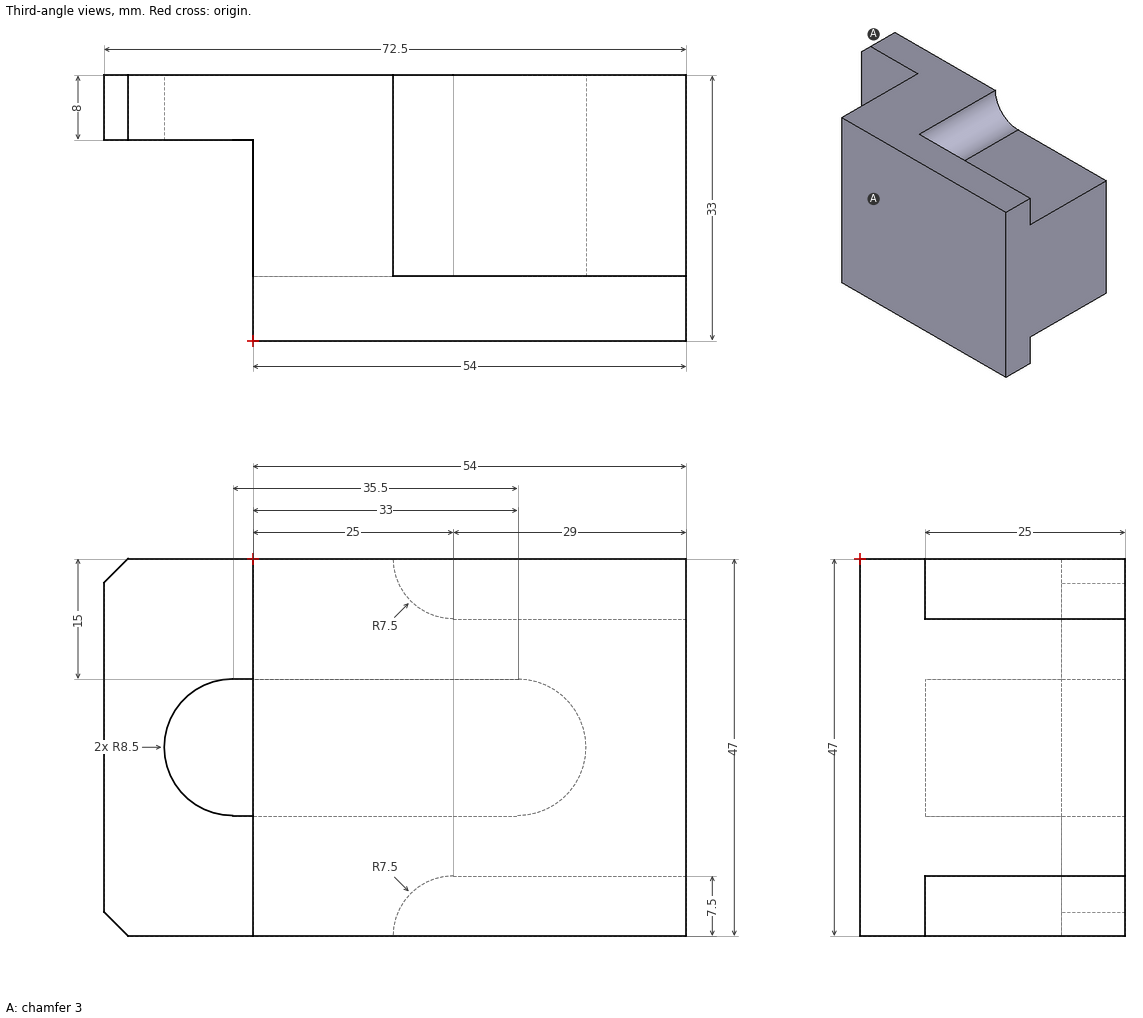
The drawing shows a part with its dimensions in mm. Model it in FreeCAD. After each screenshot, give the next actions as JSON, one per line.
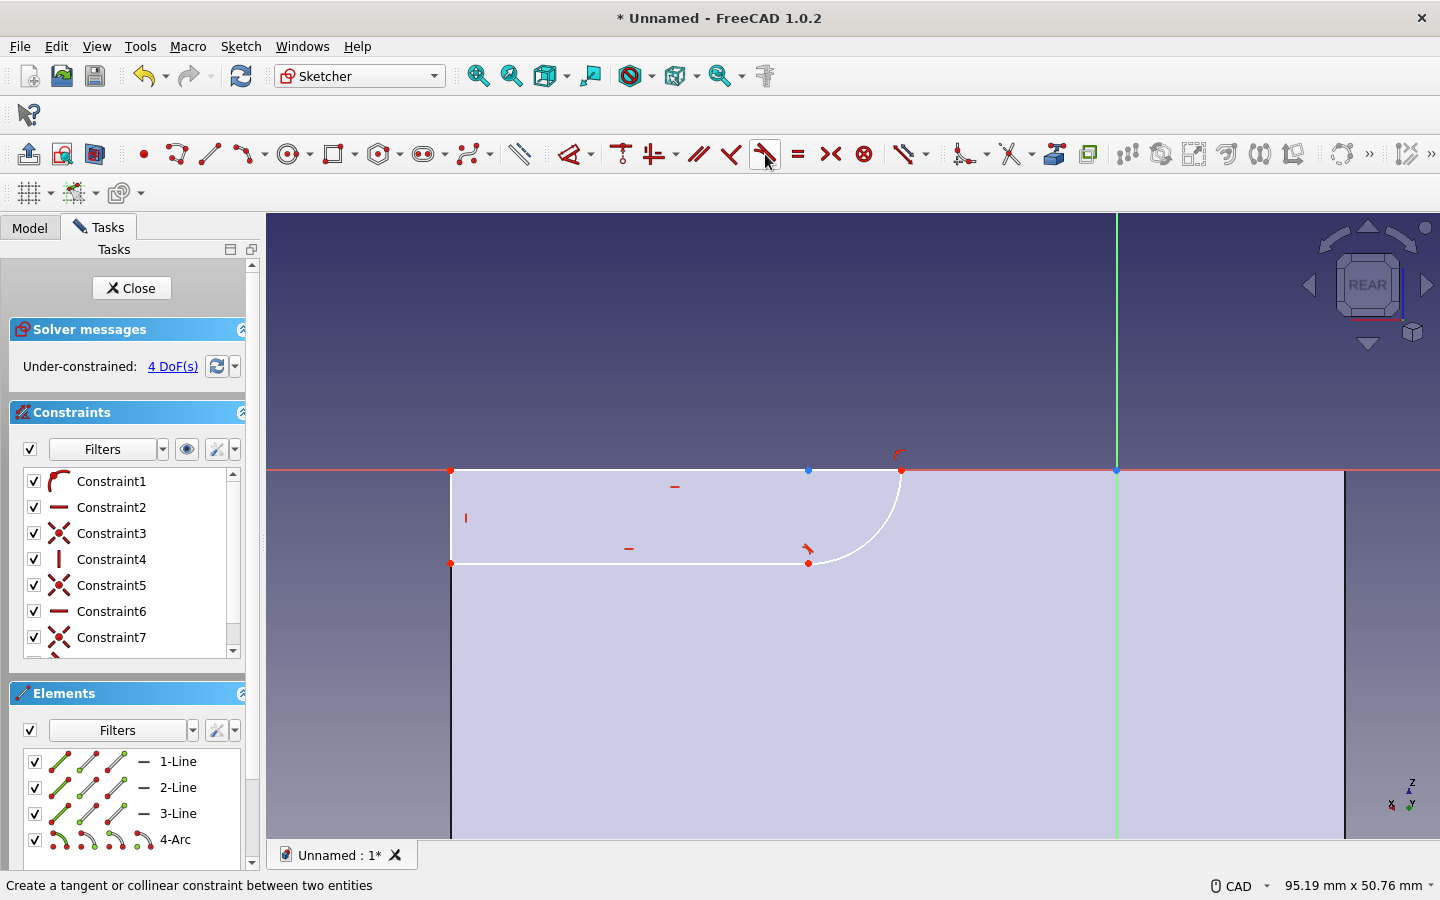
{"action": "left_click", "coordinate": [808, 471]}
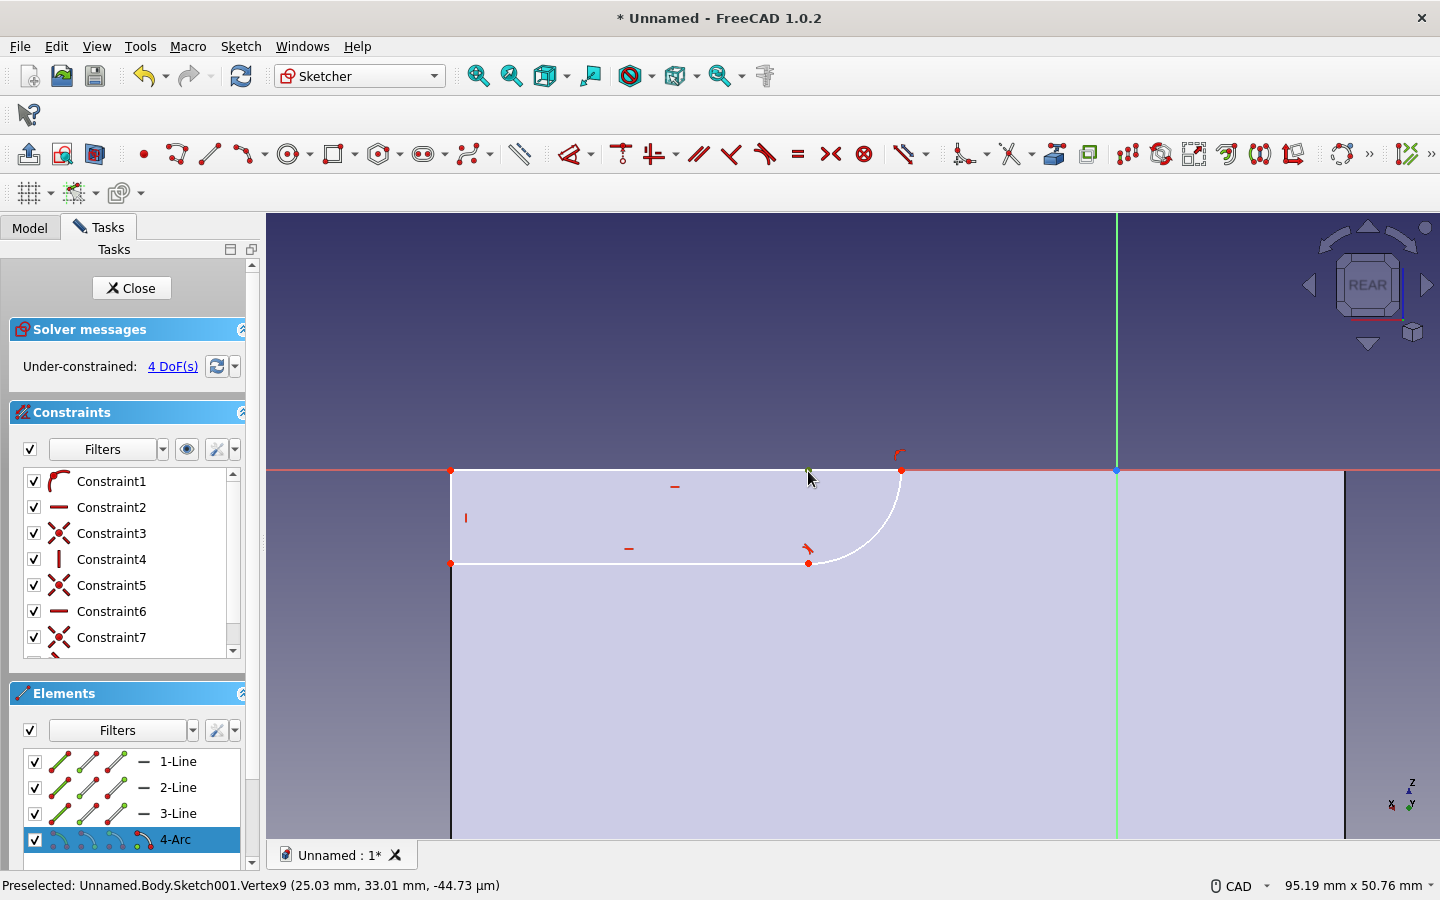
{"action": "left_click", "coordinate": [364, 470]}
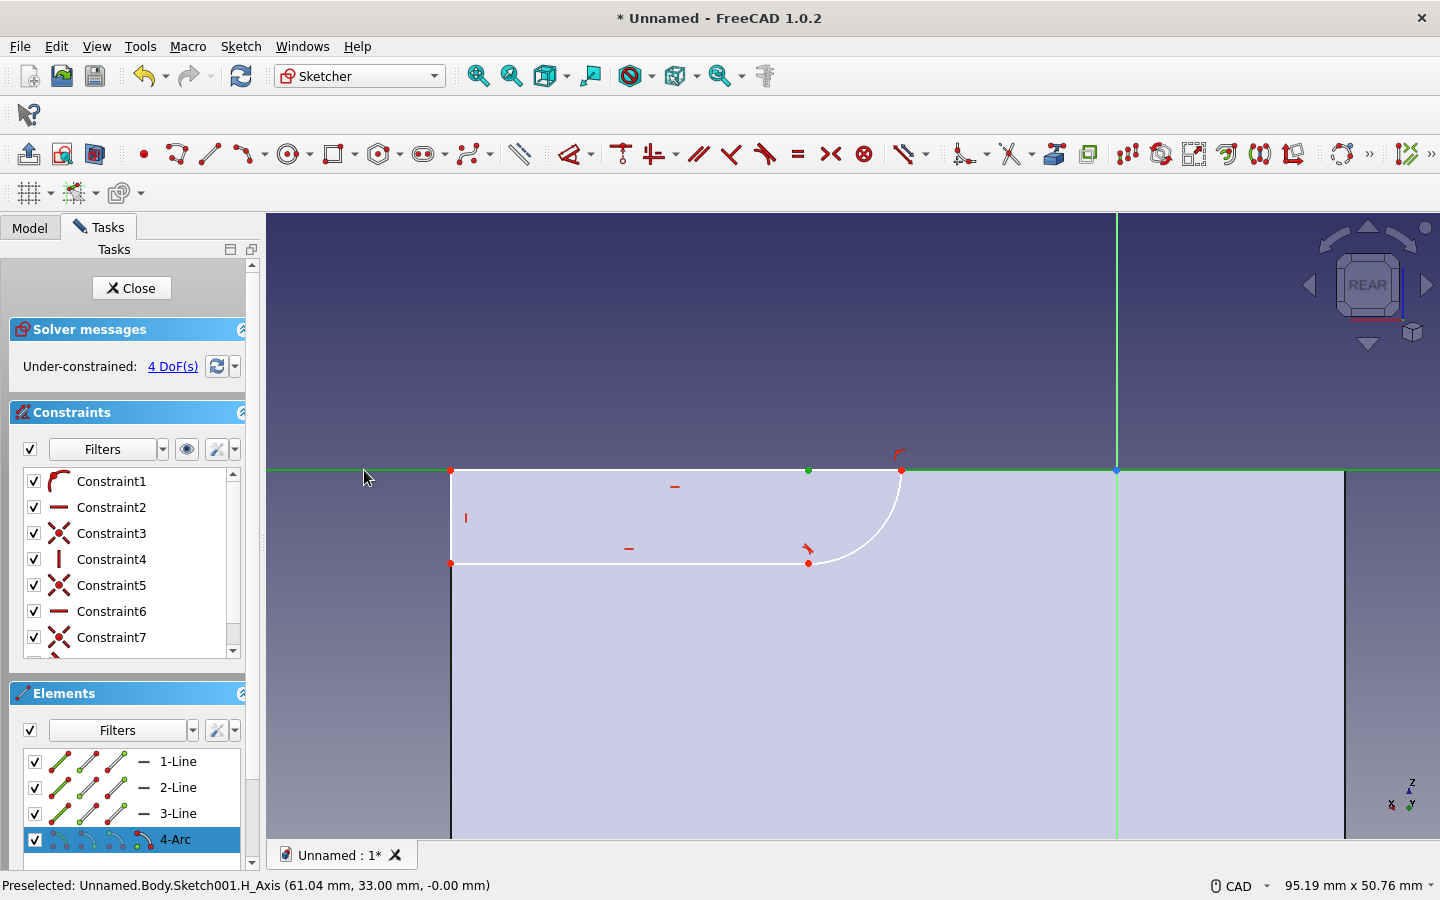
{"action": "key", "text": "c"}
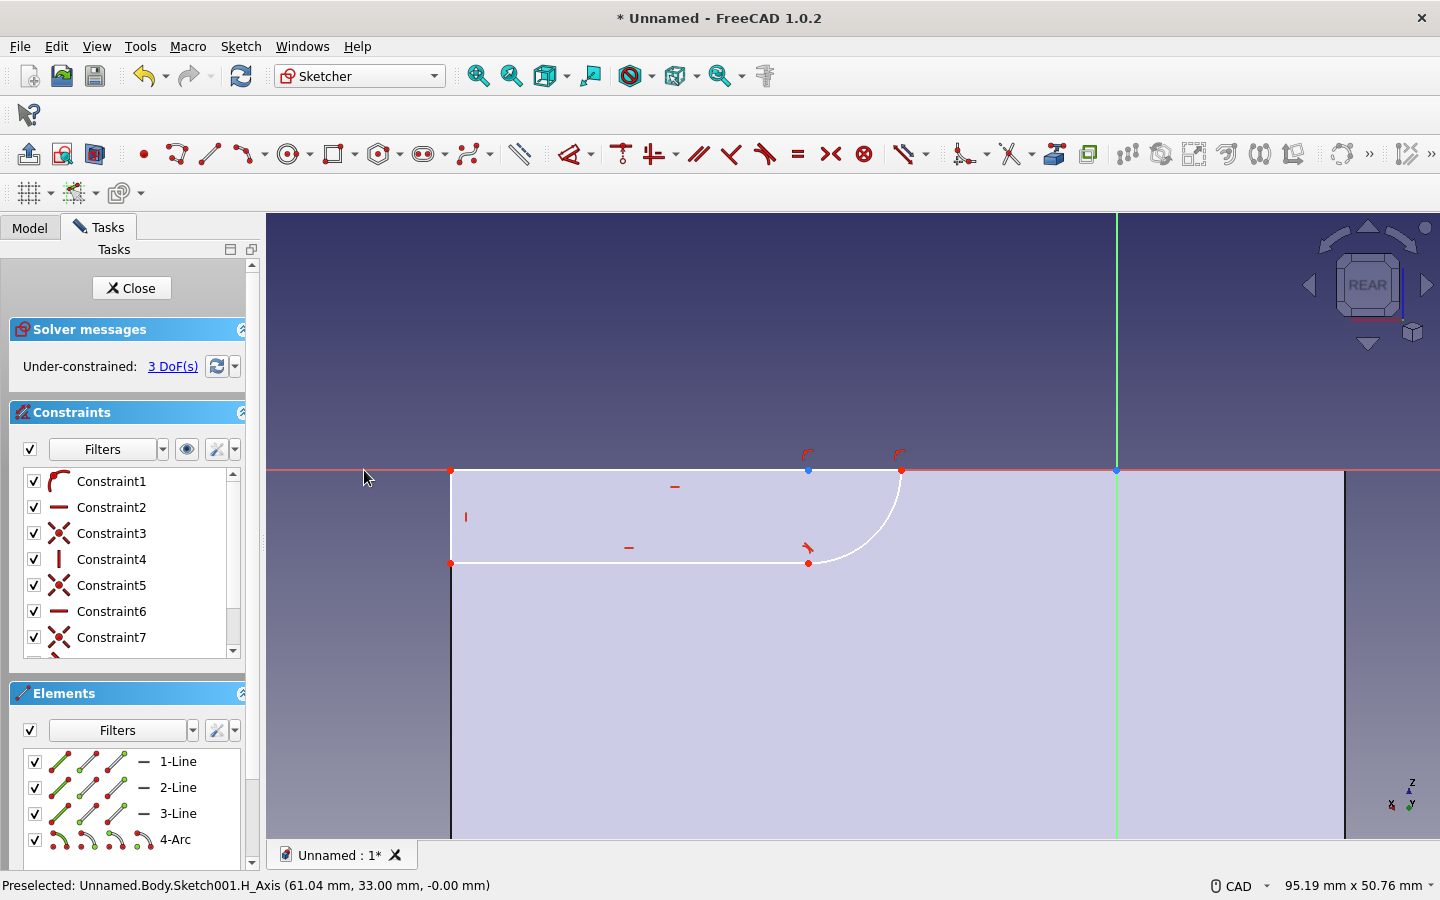
{"action": "key", "text": "d"}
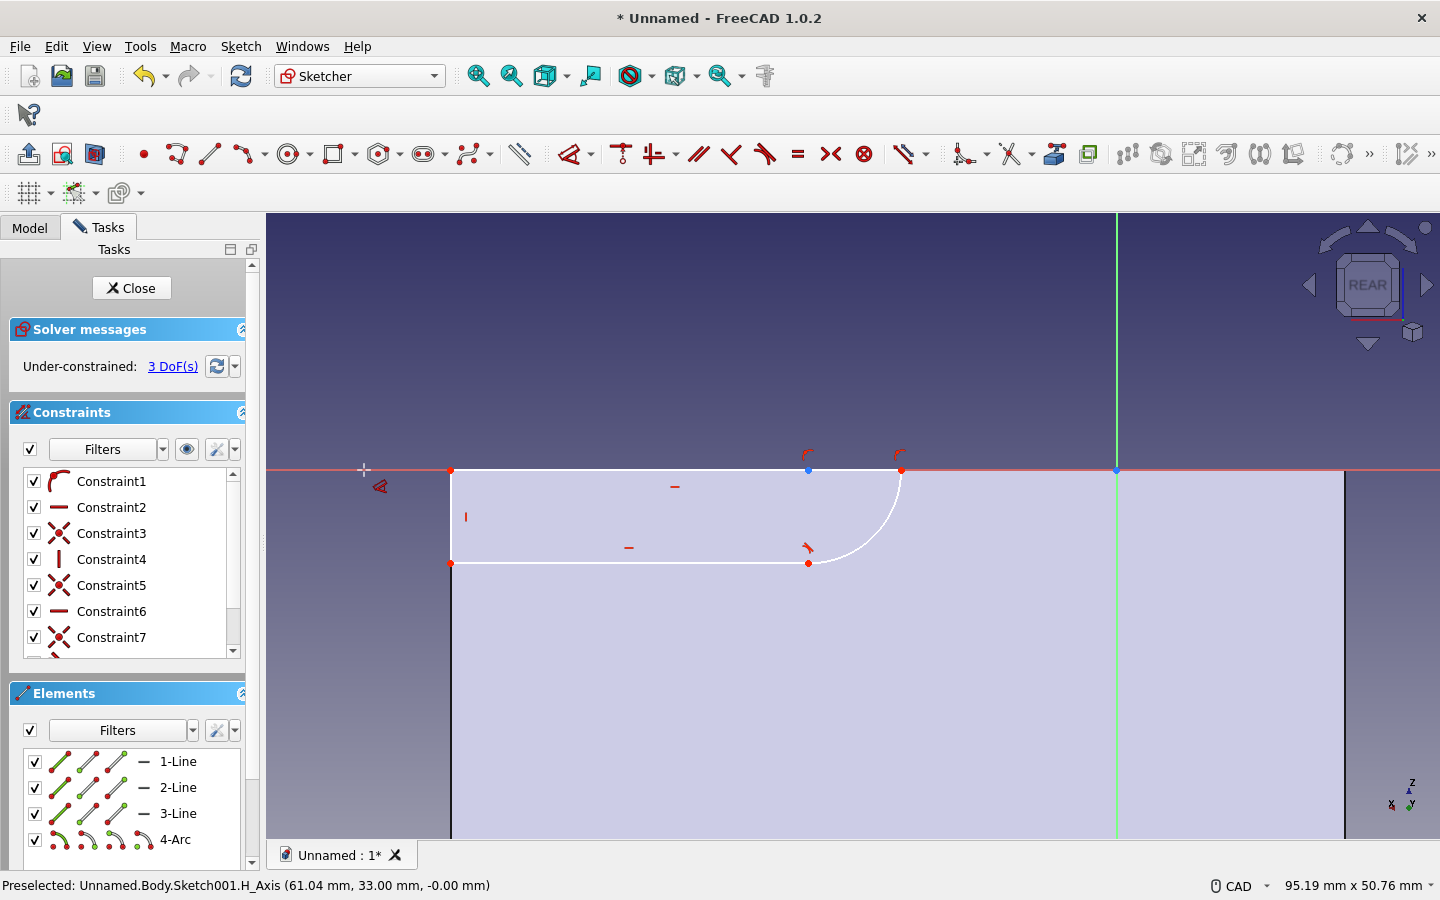
{"action": "left_click", "coordinate": [850, 553]}
{"action": "left_click", "coordinate": [865, 582]}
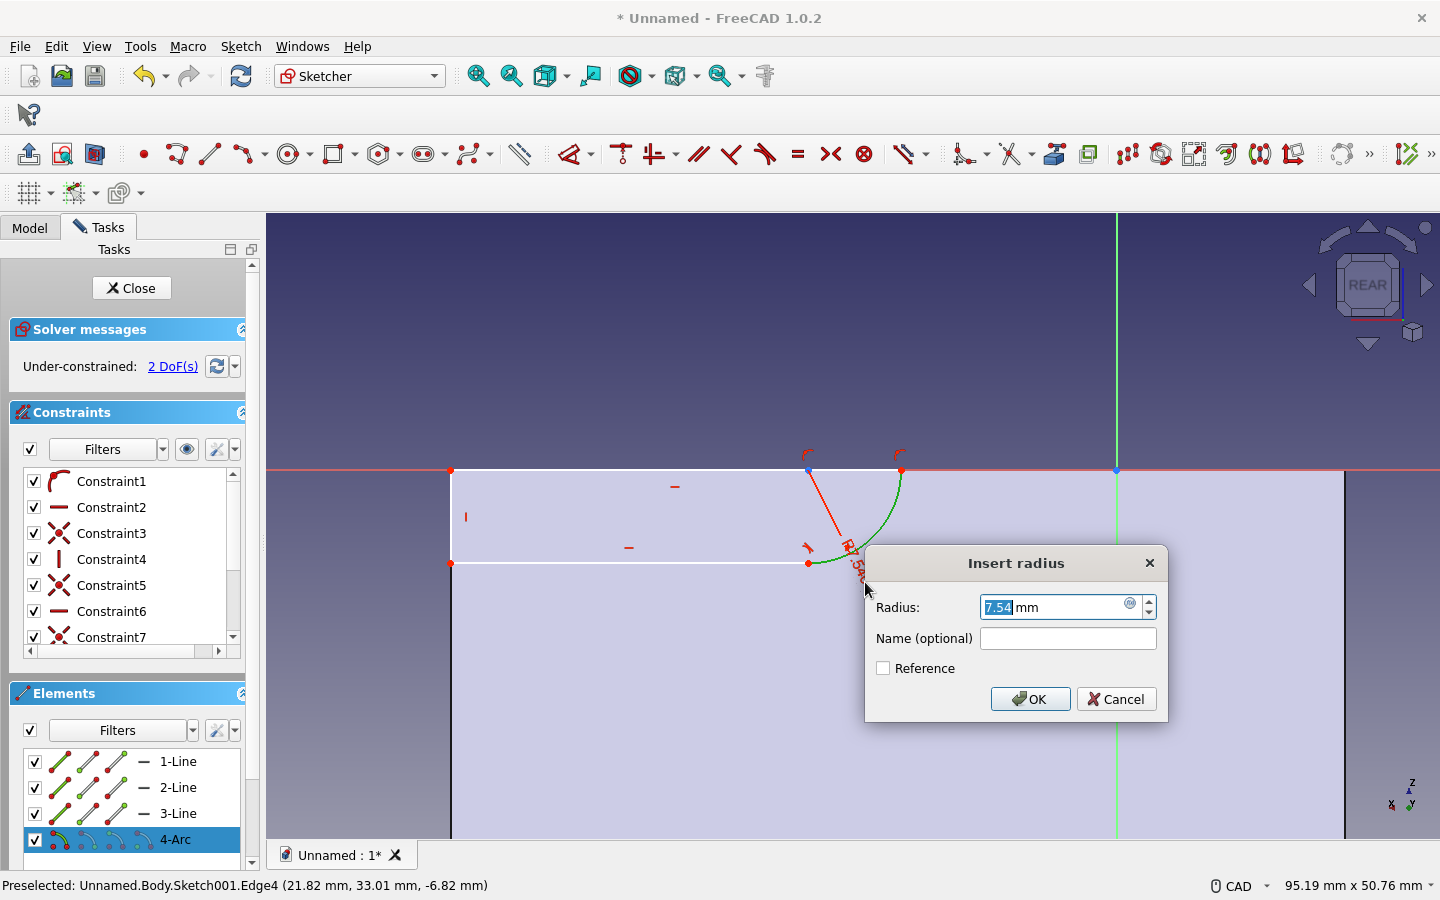
{"action": "type", "text": "7.5"}
{"action": "key", "text": "Return"}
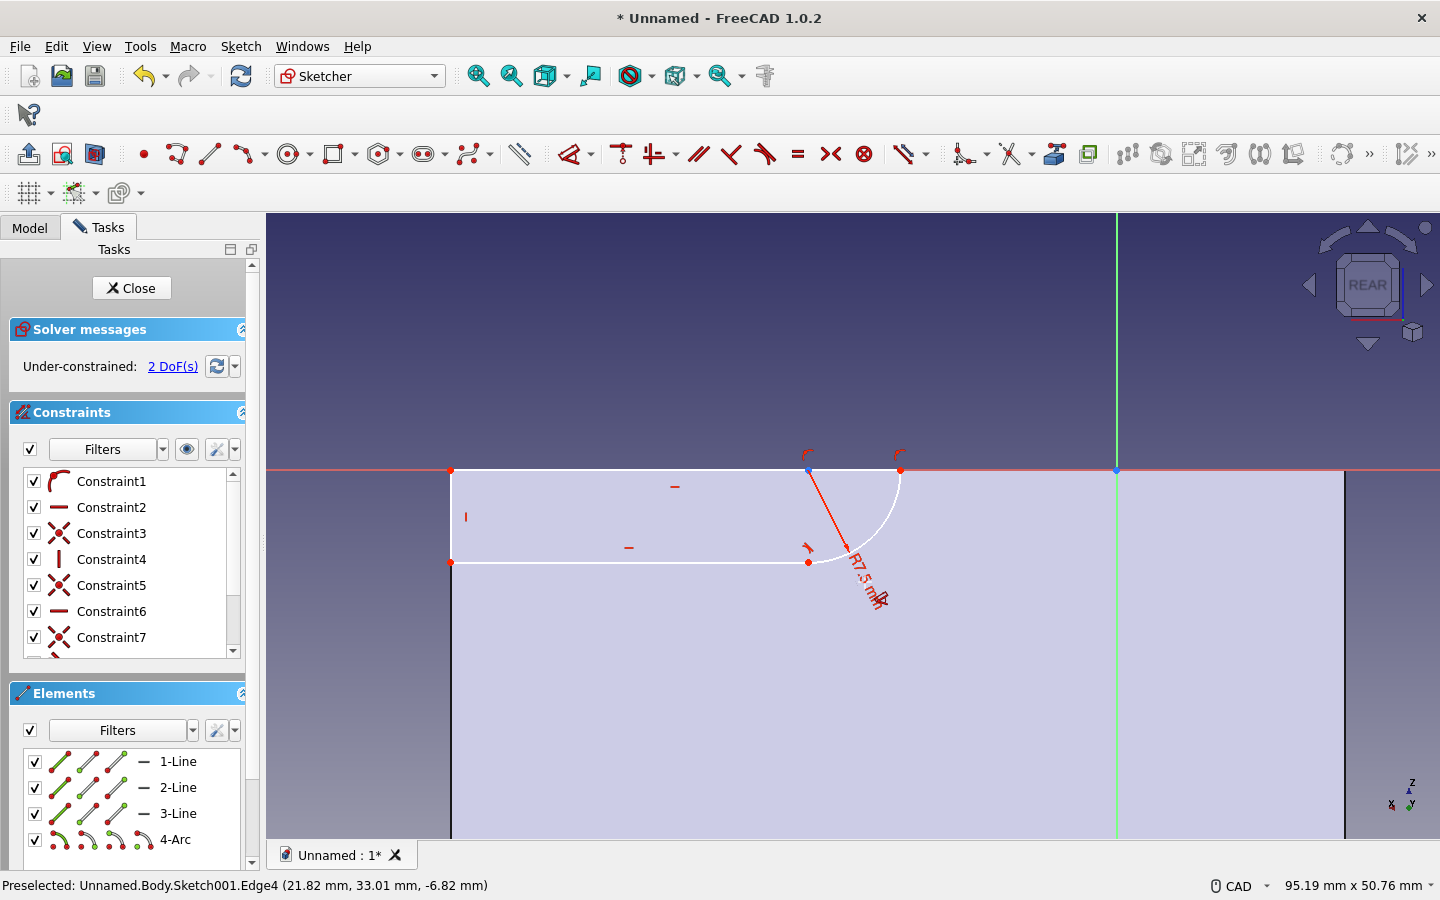
{"action": "left_click", "coordinate": [558, 563]}
{"action": "left_click", "coordinate": [630, 597]}